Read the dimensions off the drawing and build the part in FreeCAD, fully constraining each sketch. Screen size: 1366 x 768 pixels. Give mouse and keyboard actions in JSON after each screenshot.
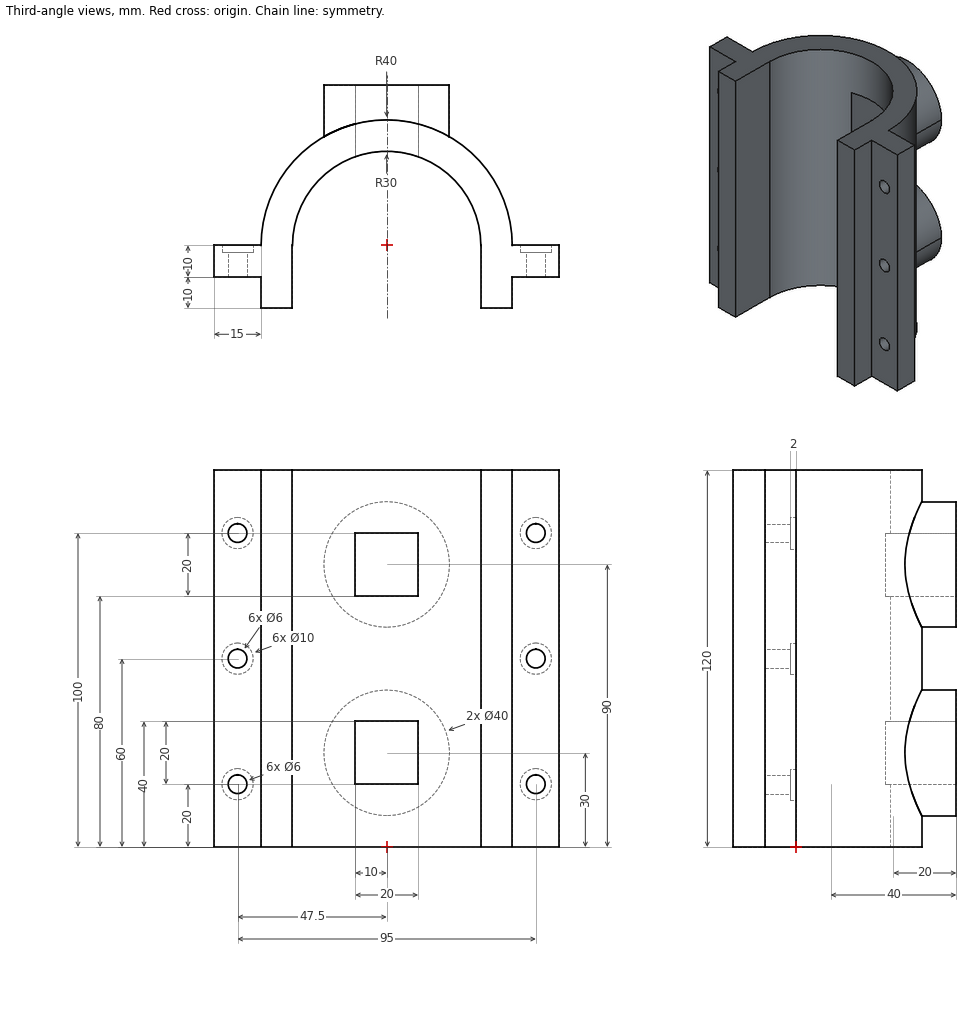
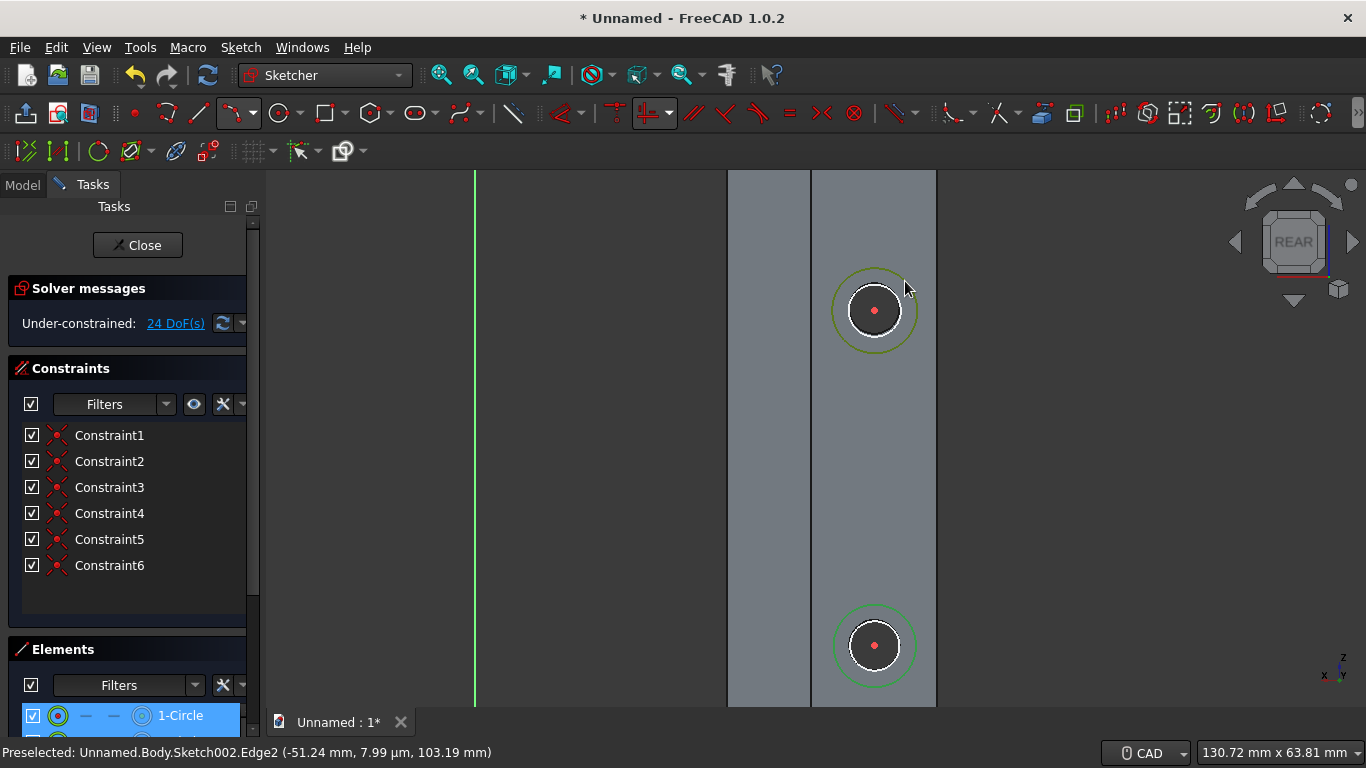
{"action": "scroll", "coordinate": [906, 282], "scroll_direction": "down", "scroll_amount": 5}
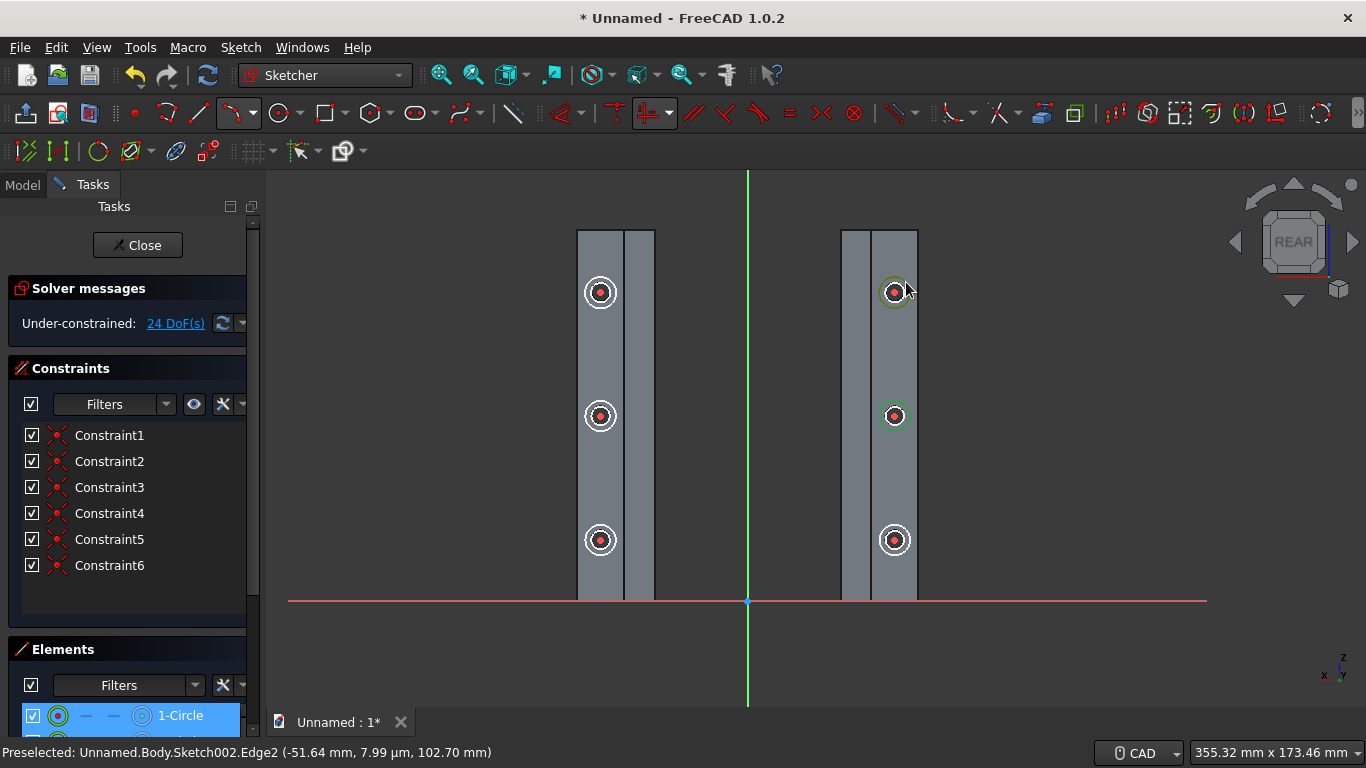
{"action": "scroll", "coordinate": [906, 529], "scroll_direction": "up", "scroll_amount": 5}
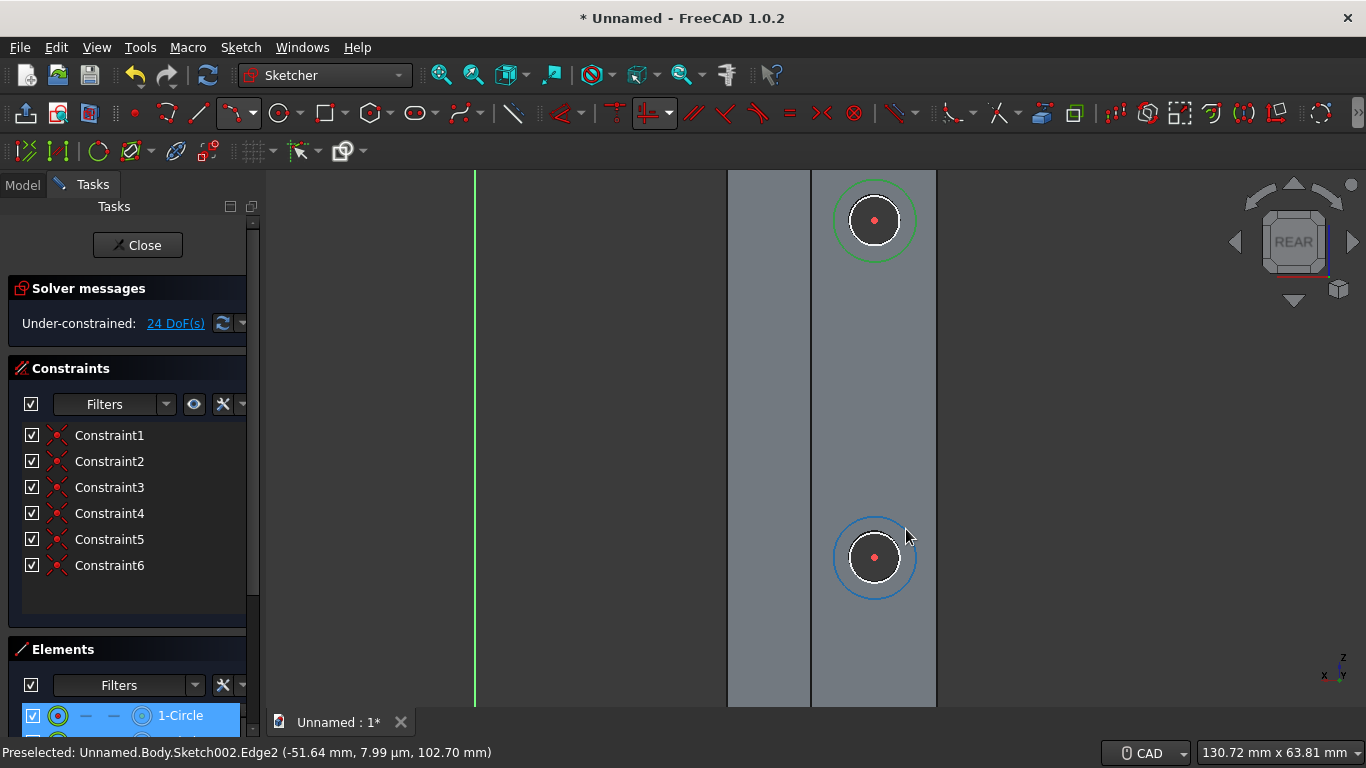
{"action": "left_click", "coordinate": [904, 529]}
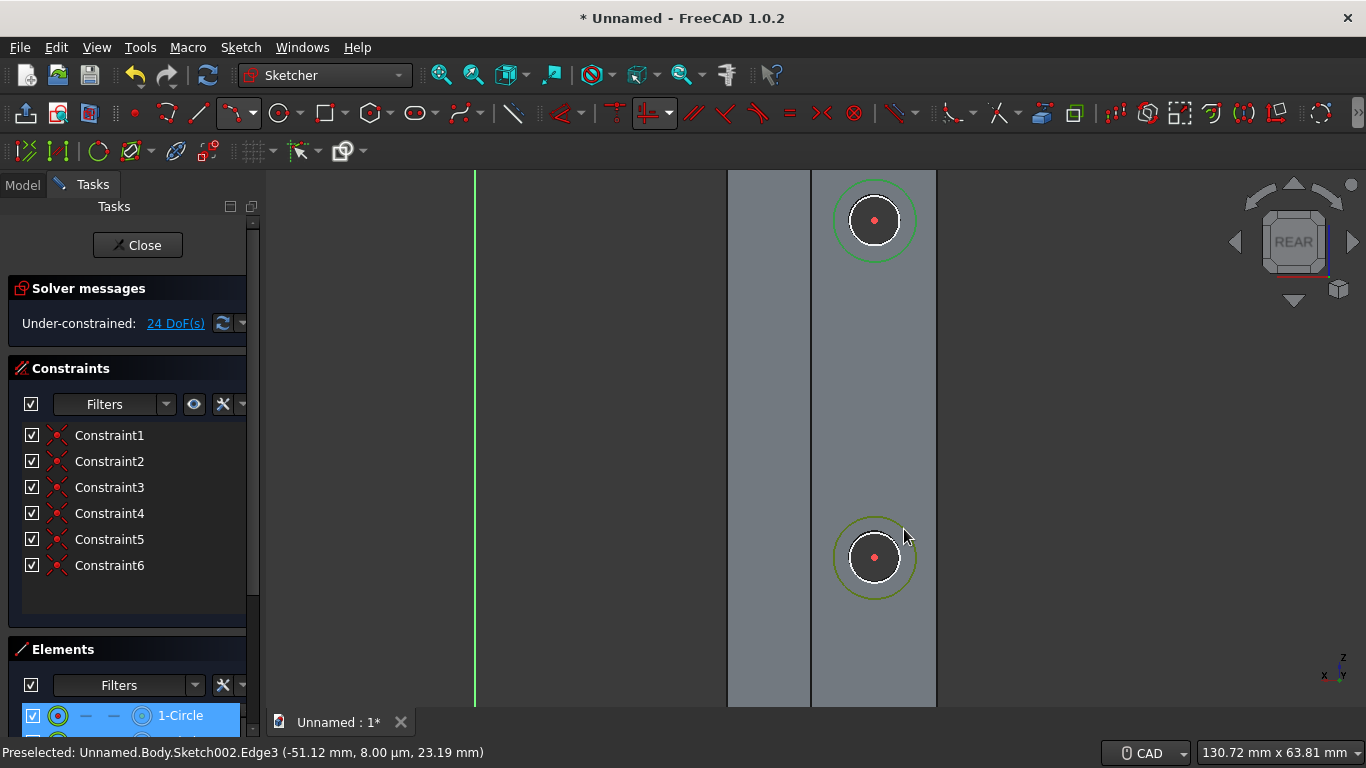
{"action": "scroll", "coordinate": [906, 529], "scroll_direction": "down", "scroll_amount": 5}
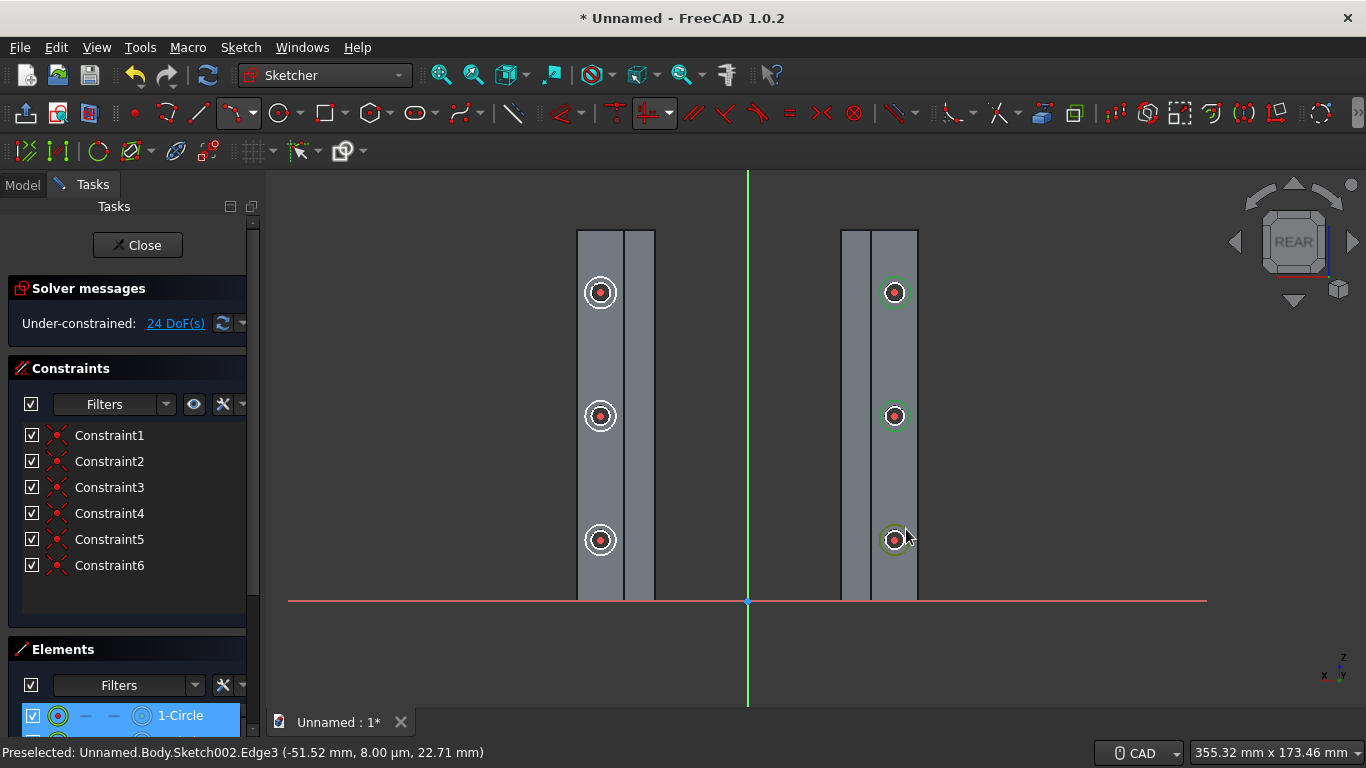
{"action": "scroll", "coordinate": [611, 529], "scroll_direction": "up", "scroll_amount": 5}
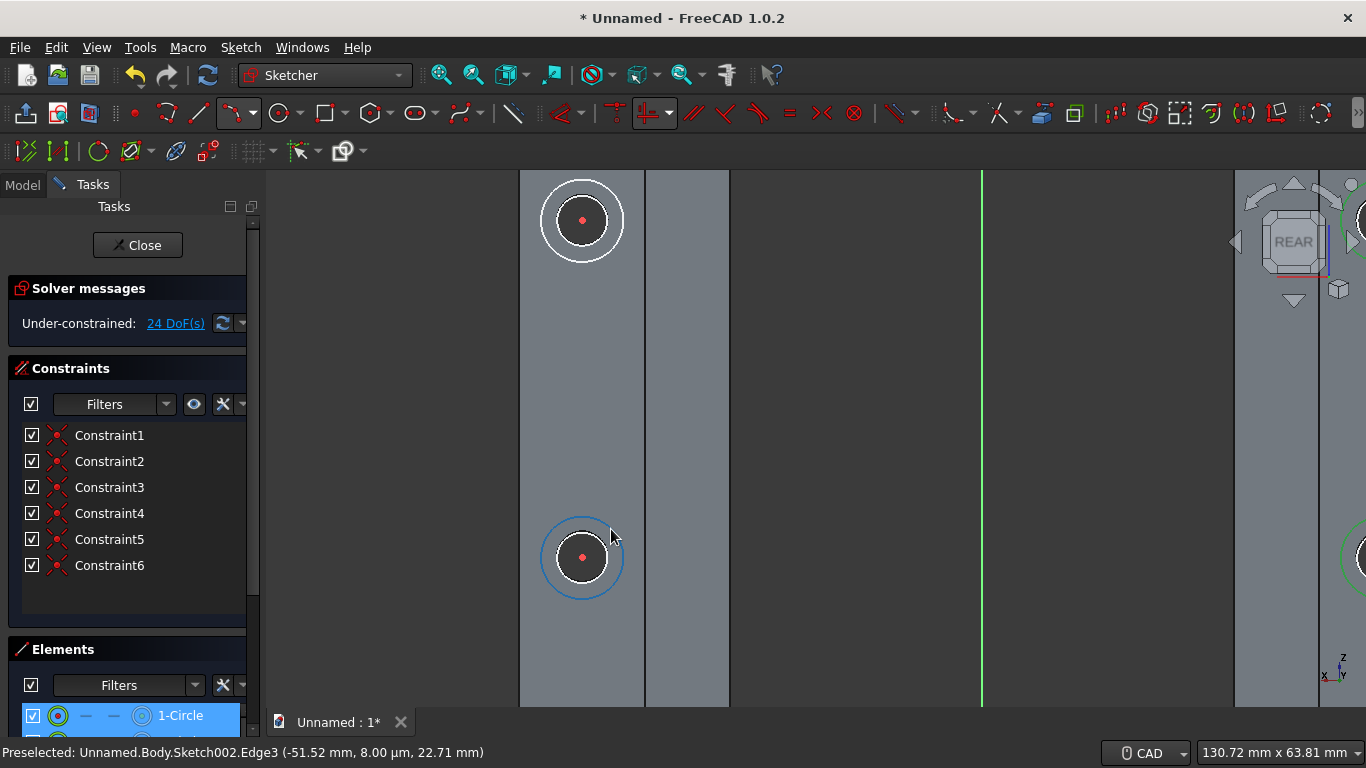
{"action": "left_click", "coordinate": [611, 529]}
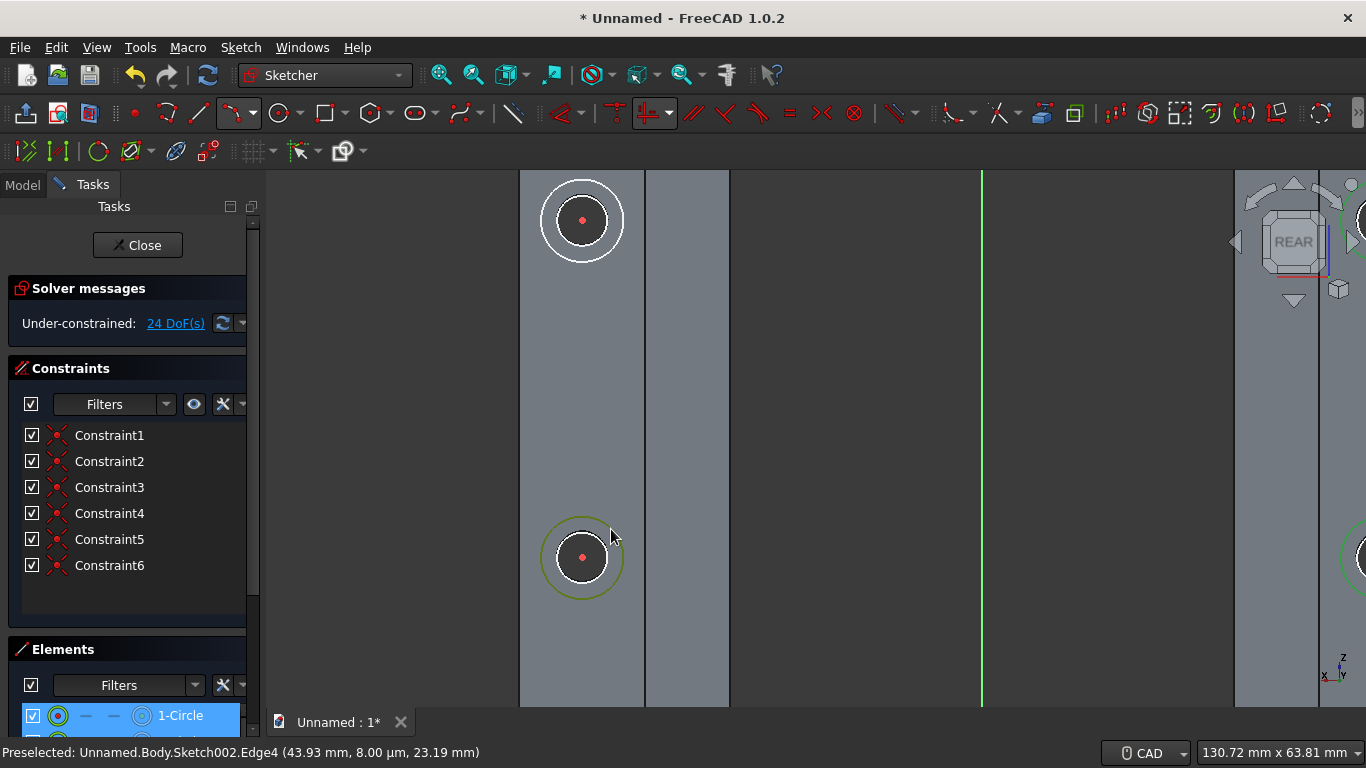
{"action": "left_click", "coordinate": [553, 250]}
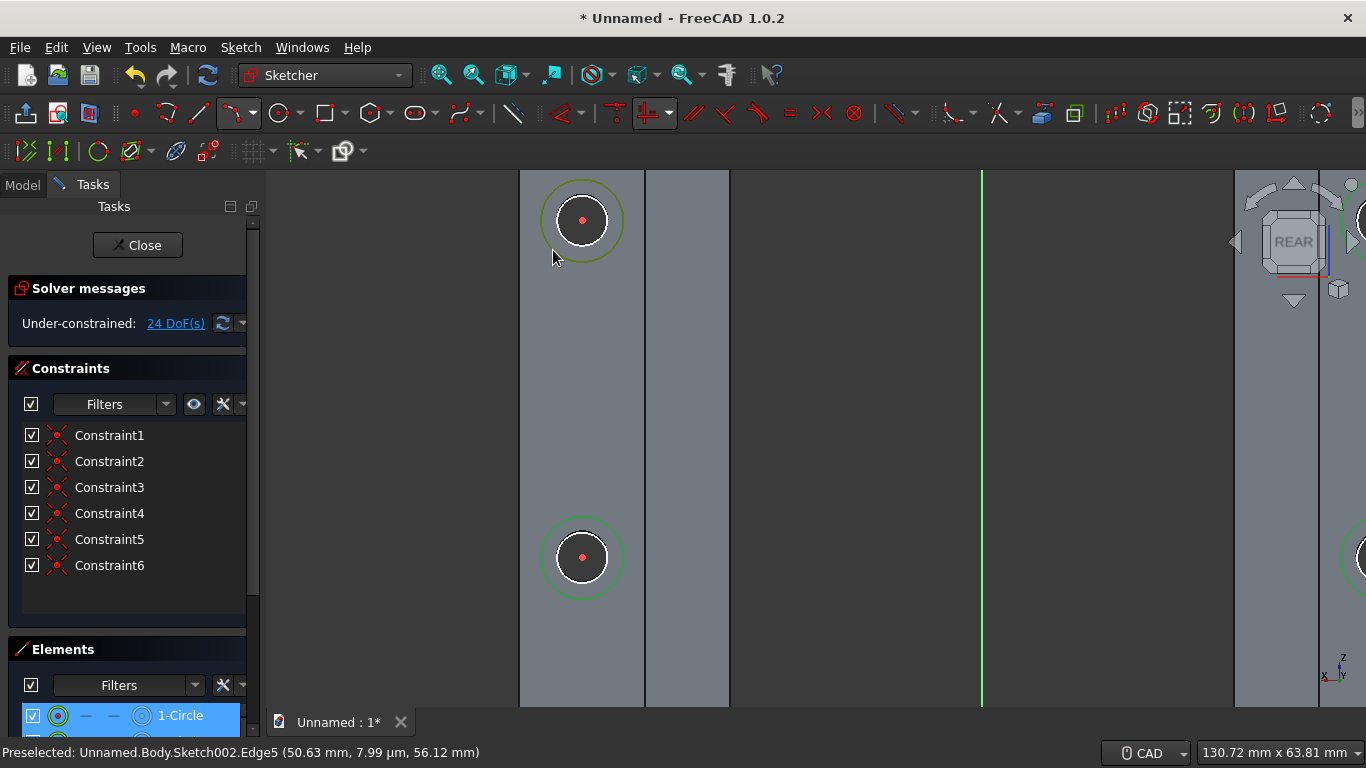
{"action": "scroll", "coordinate": [611, 529], "scroll_direction": "down", "scroll_amount": 5}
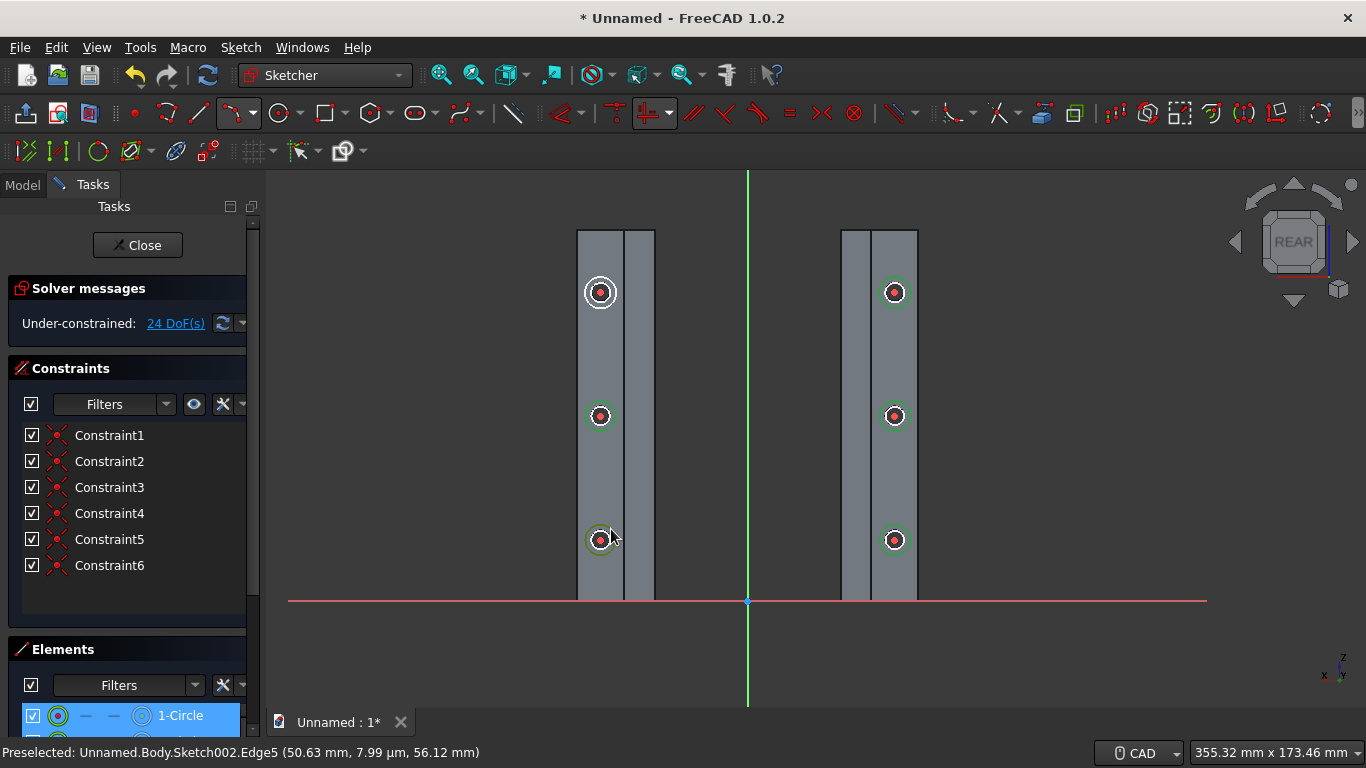
{"action": "scroll", "coordinate": [612, 282], "scroll_direction": "up", "scroll_amount": 5}